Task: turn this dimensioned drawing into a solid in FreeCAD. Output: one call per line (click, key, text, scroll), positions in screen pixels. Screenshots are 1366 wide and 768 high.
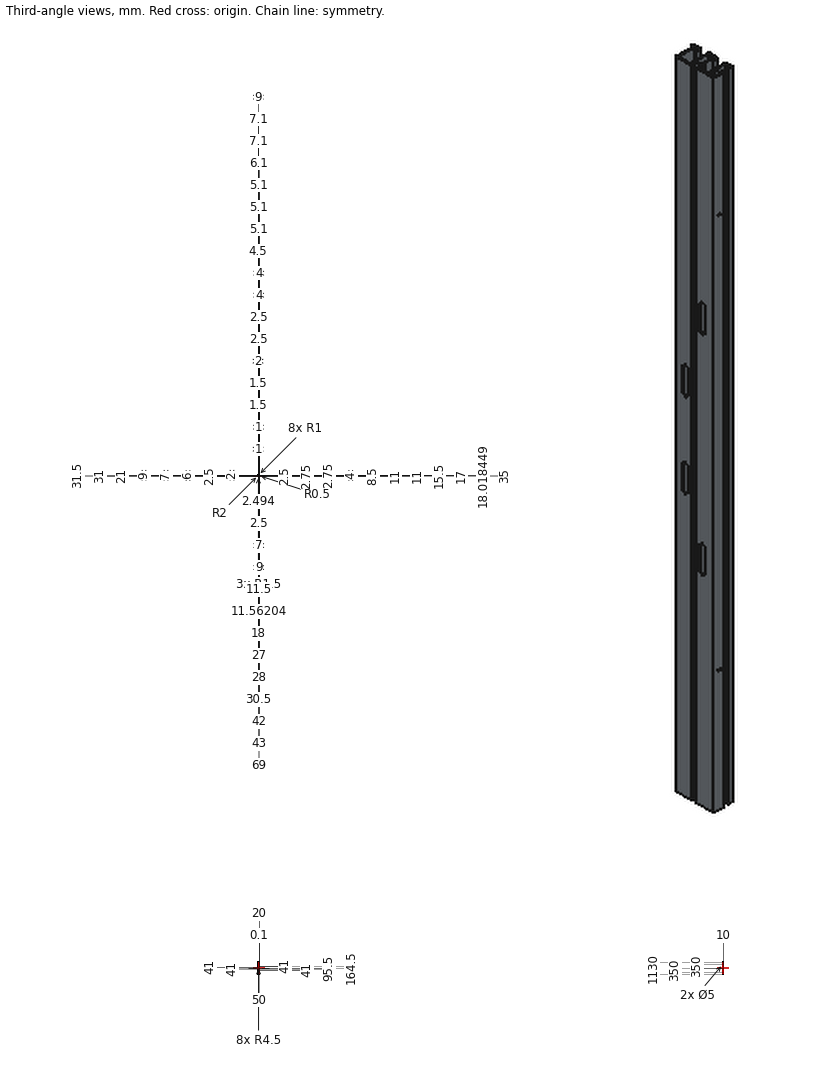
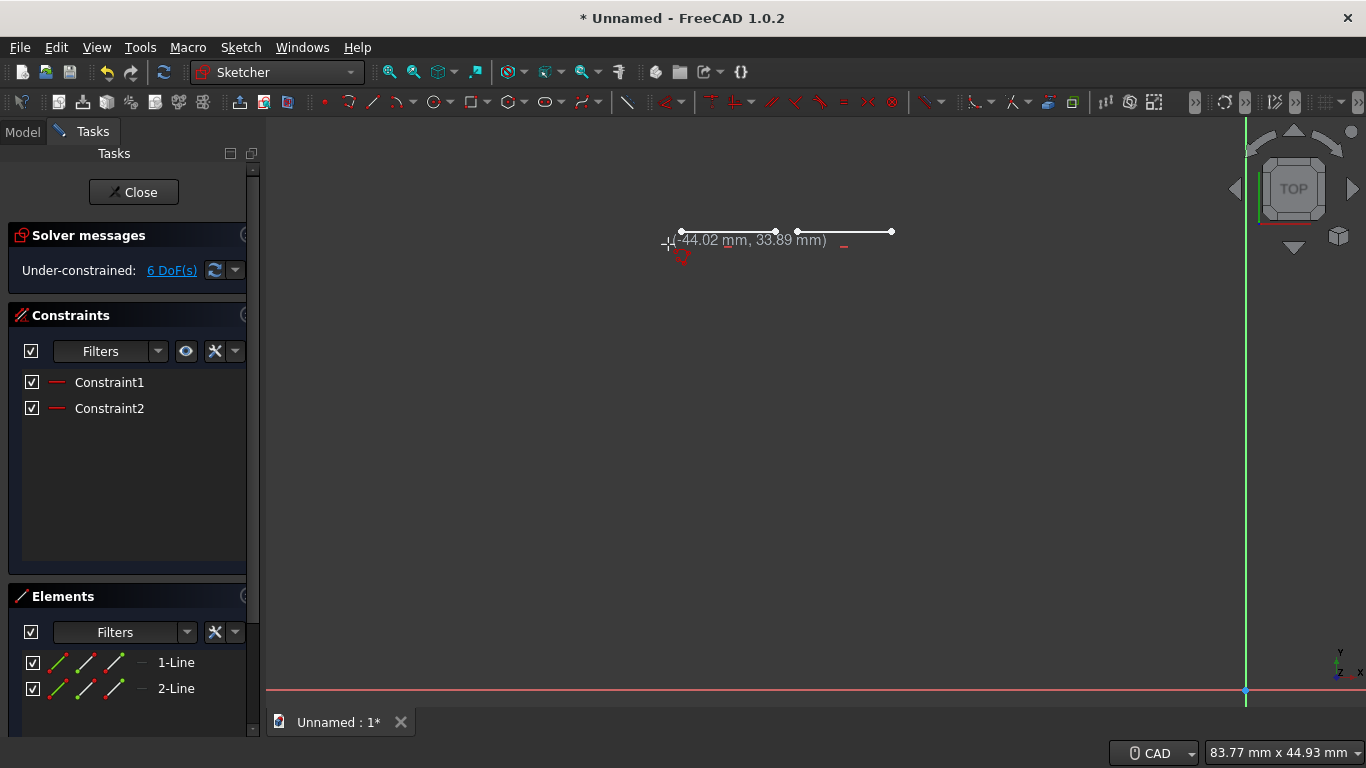
click(668, 244)
click(668, 658)
click(432, 658)
right_click(432, 658)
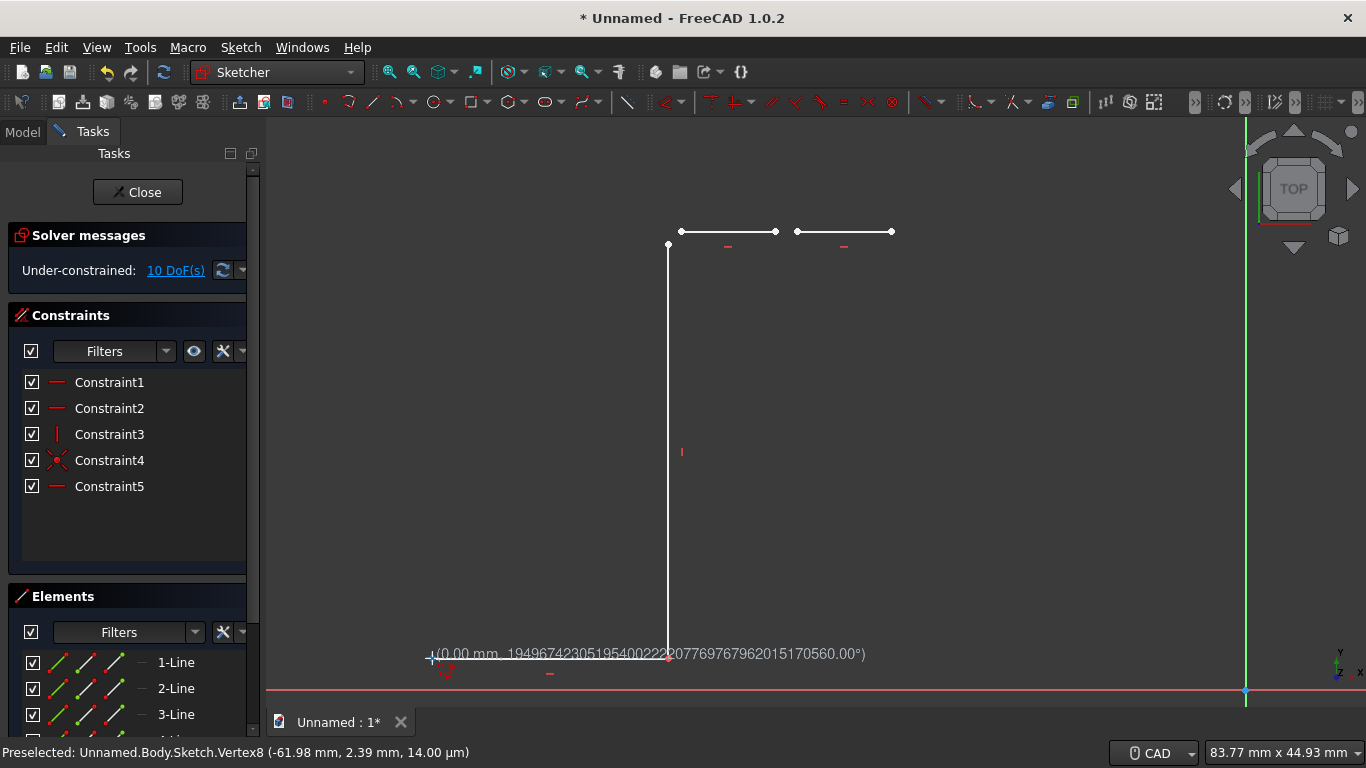
key(g)
key(l)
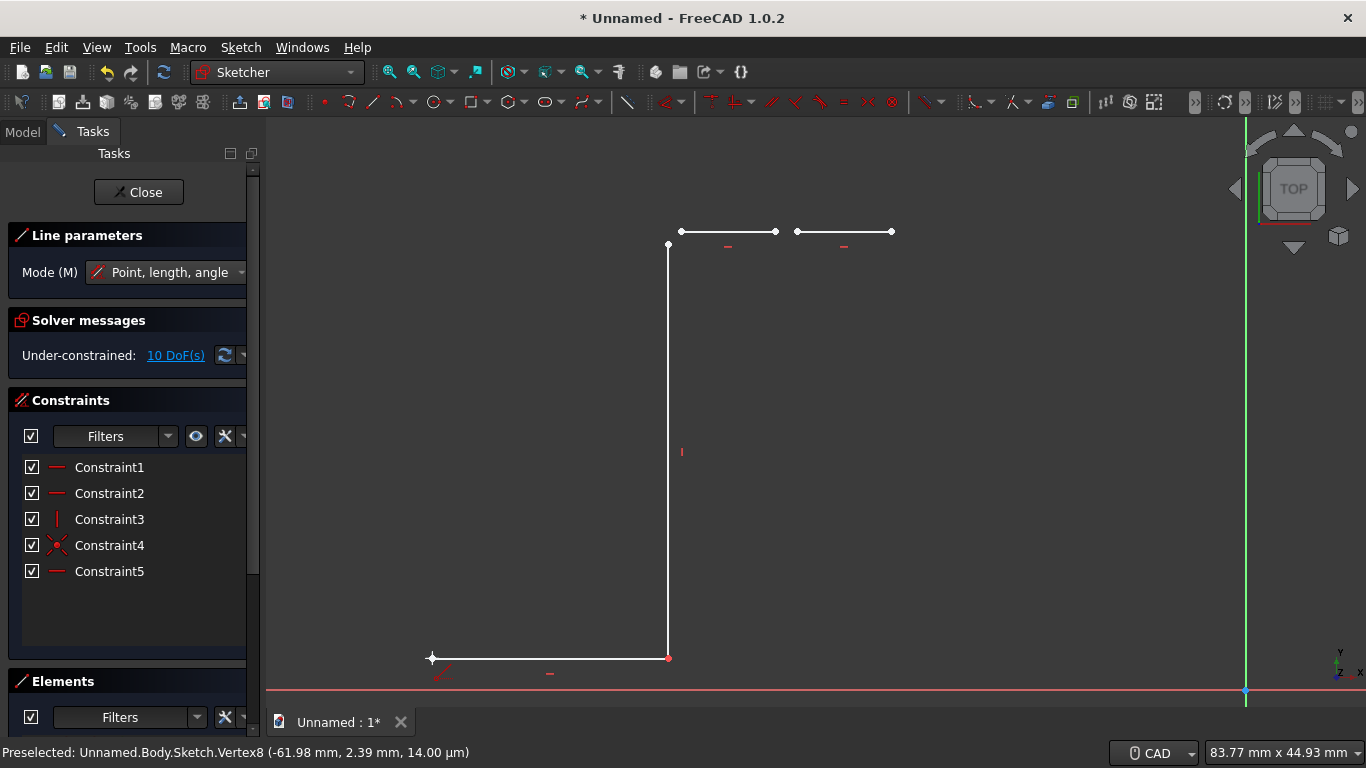
click(406, 631)
click(406, 283)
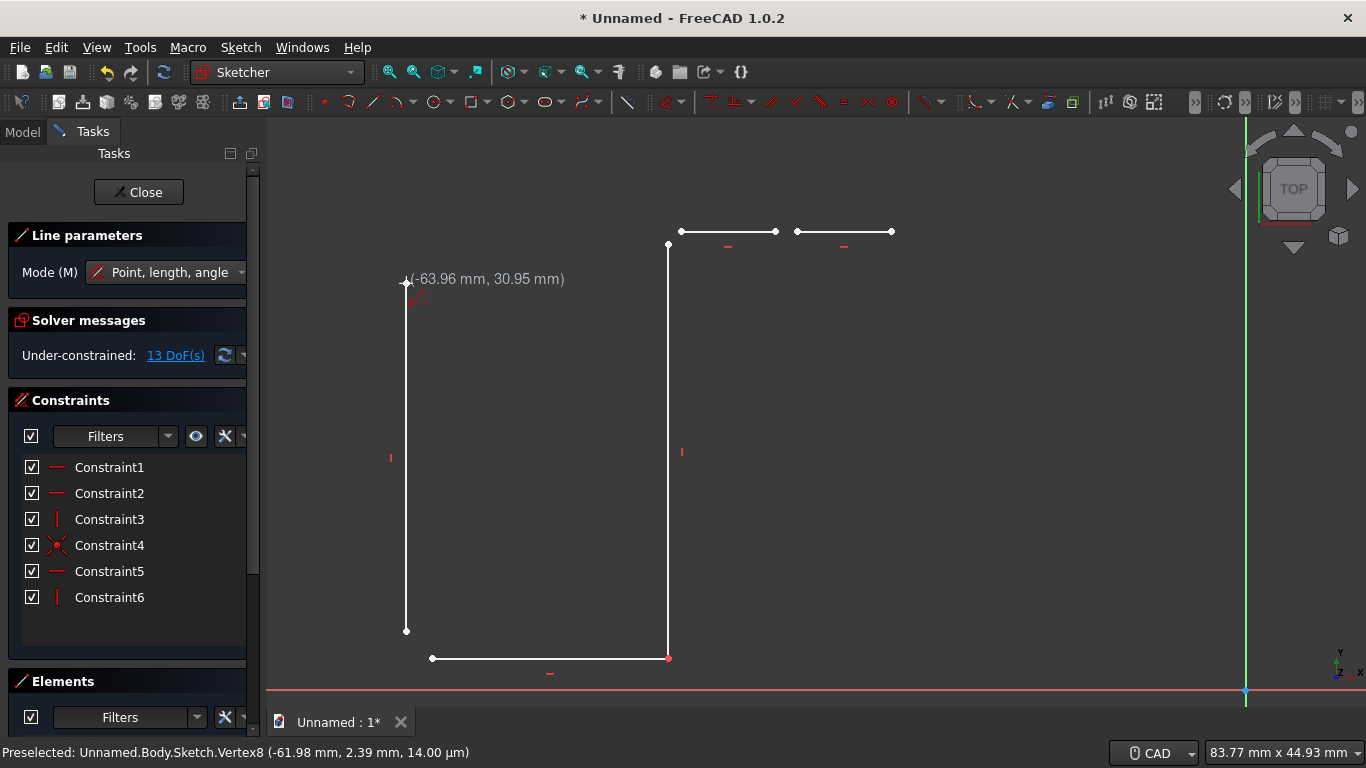
click(350, 102)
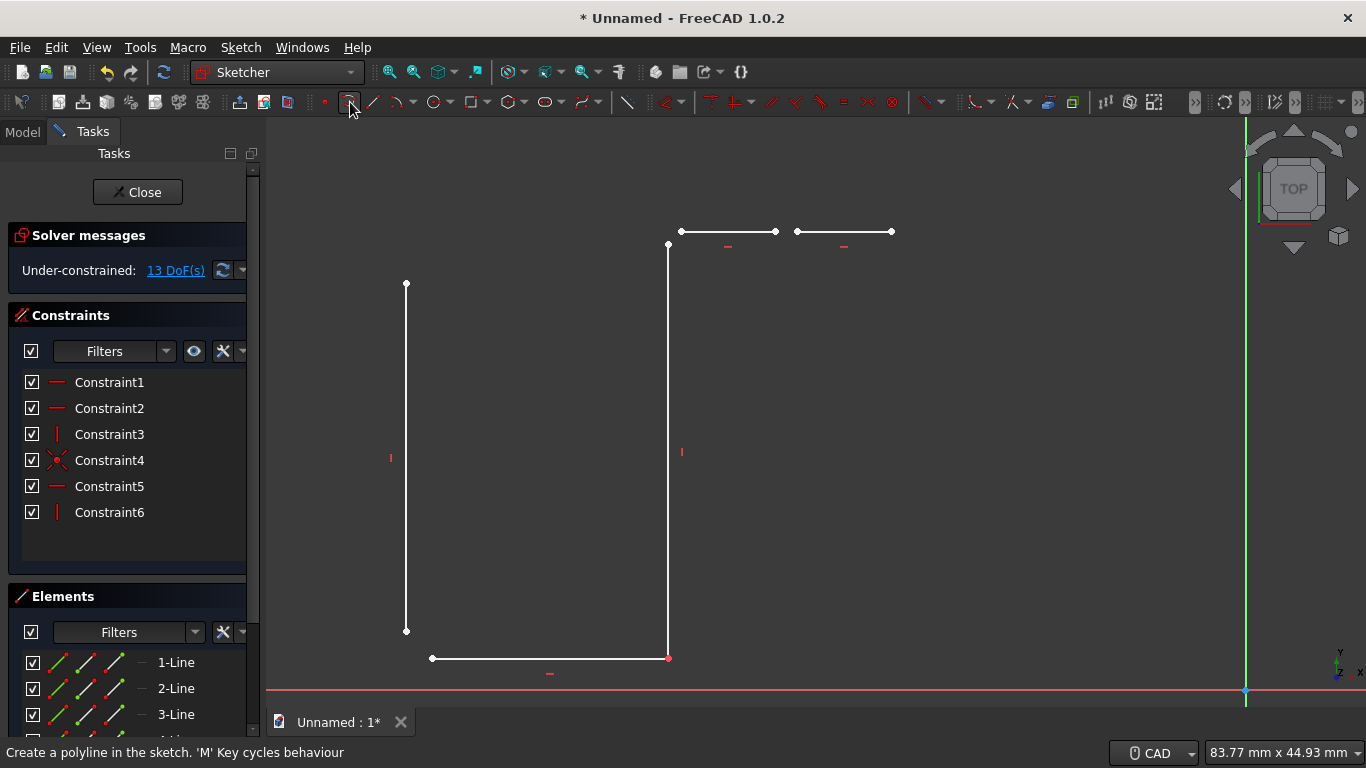
click(419, 270)
click(478, 270)
click(491, 362)
click(511, 362)
click(511, 244)
right_click(511, 244)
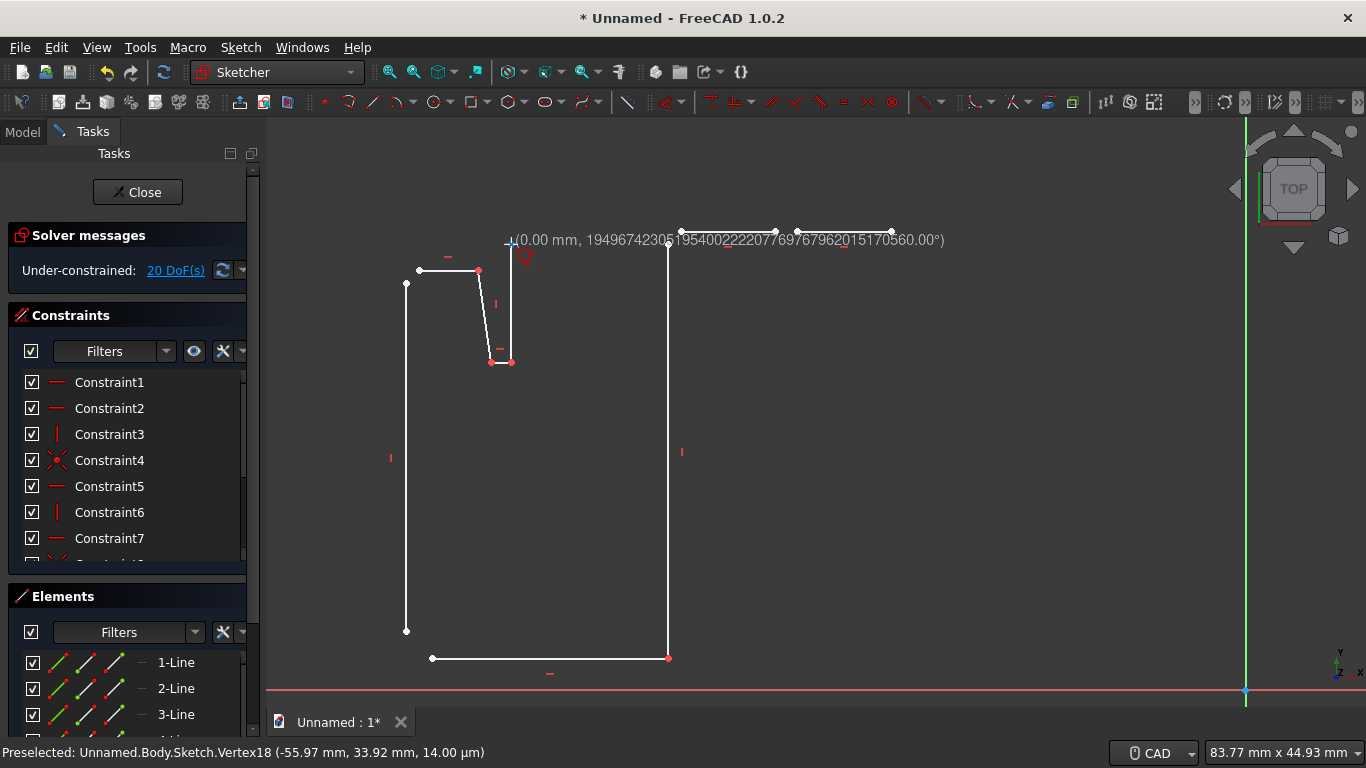
key(g)
key(l)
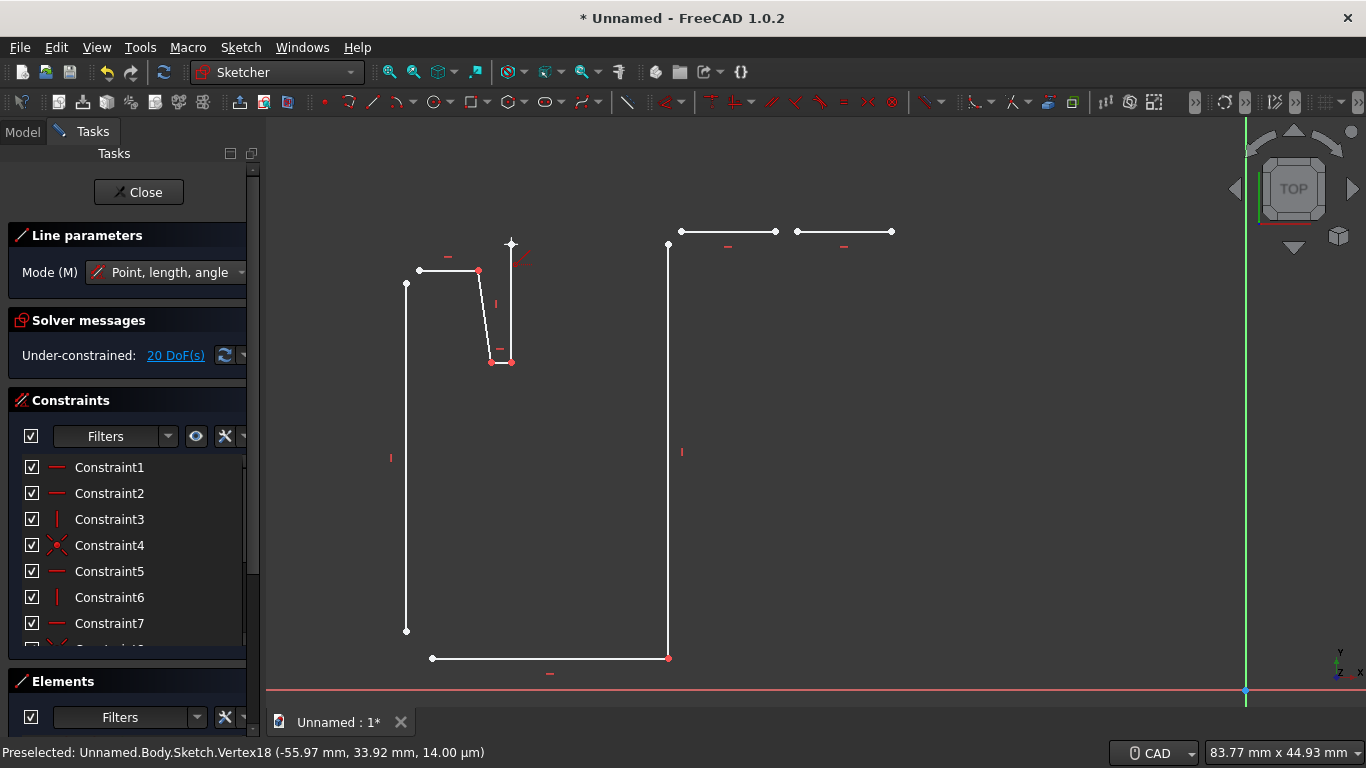
click(497, 231)
click(430, 231)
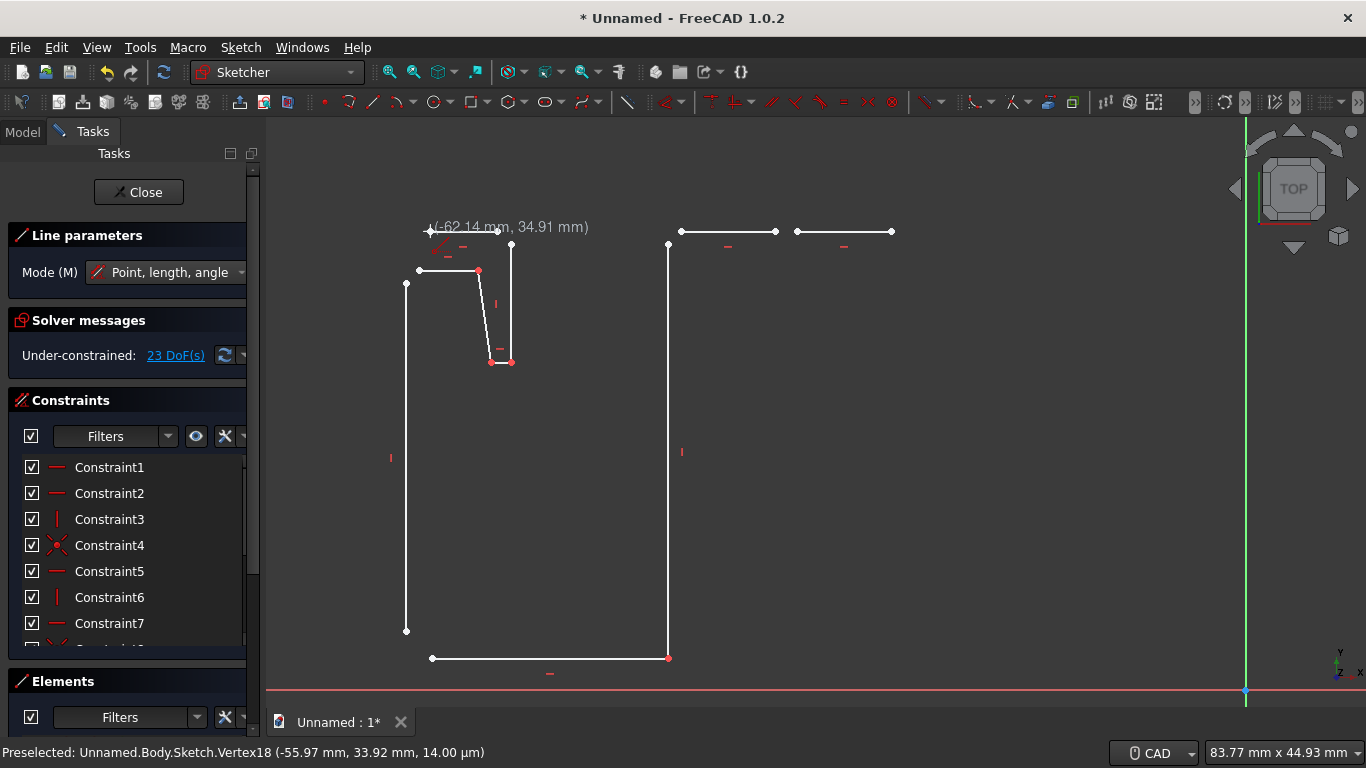
click(407, 231)
click(340, 231)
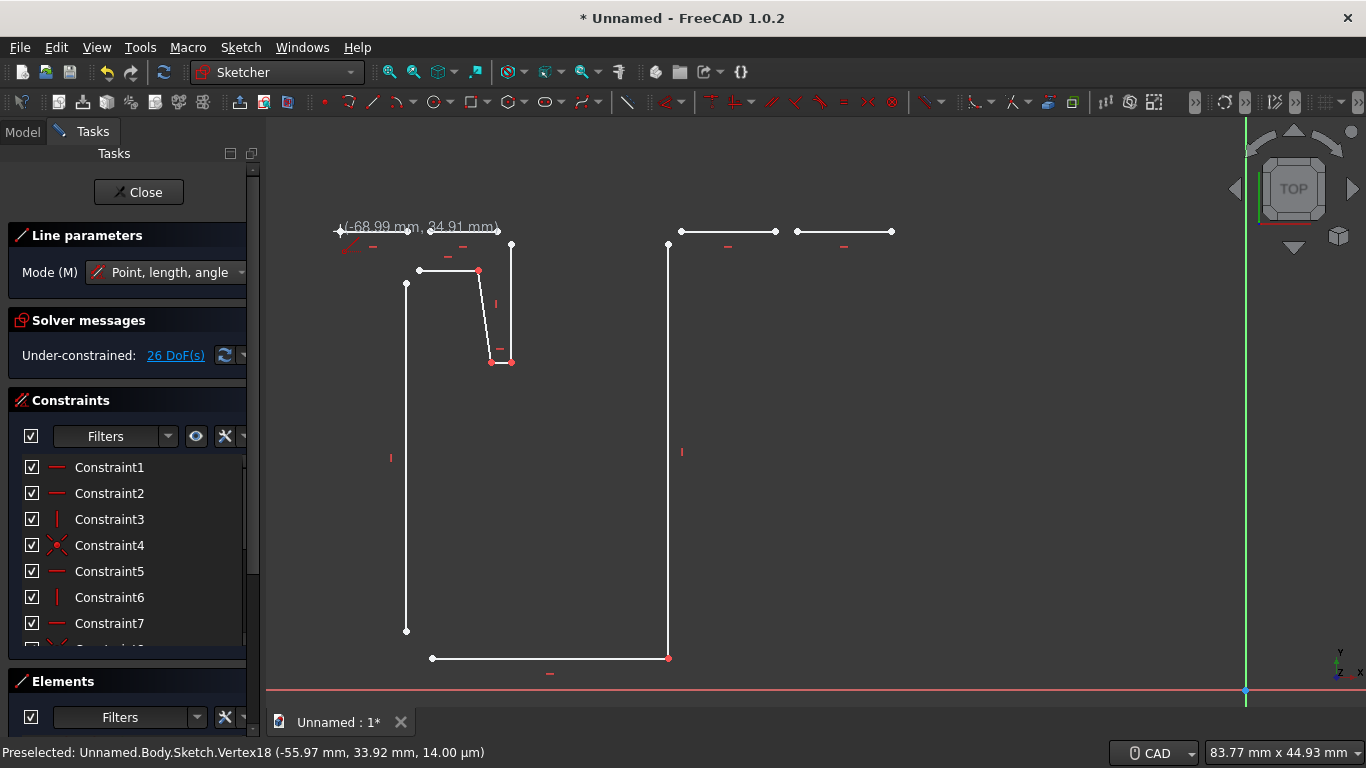
key(g)
key(m)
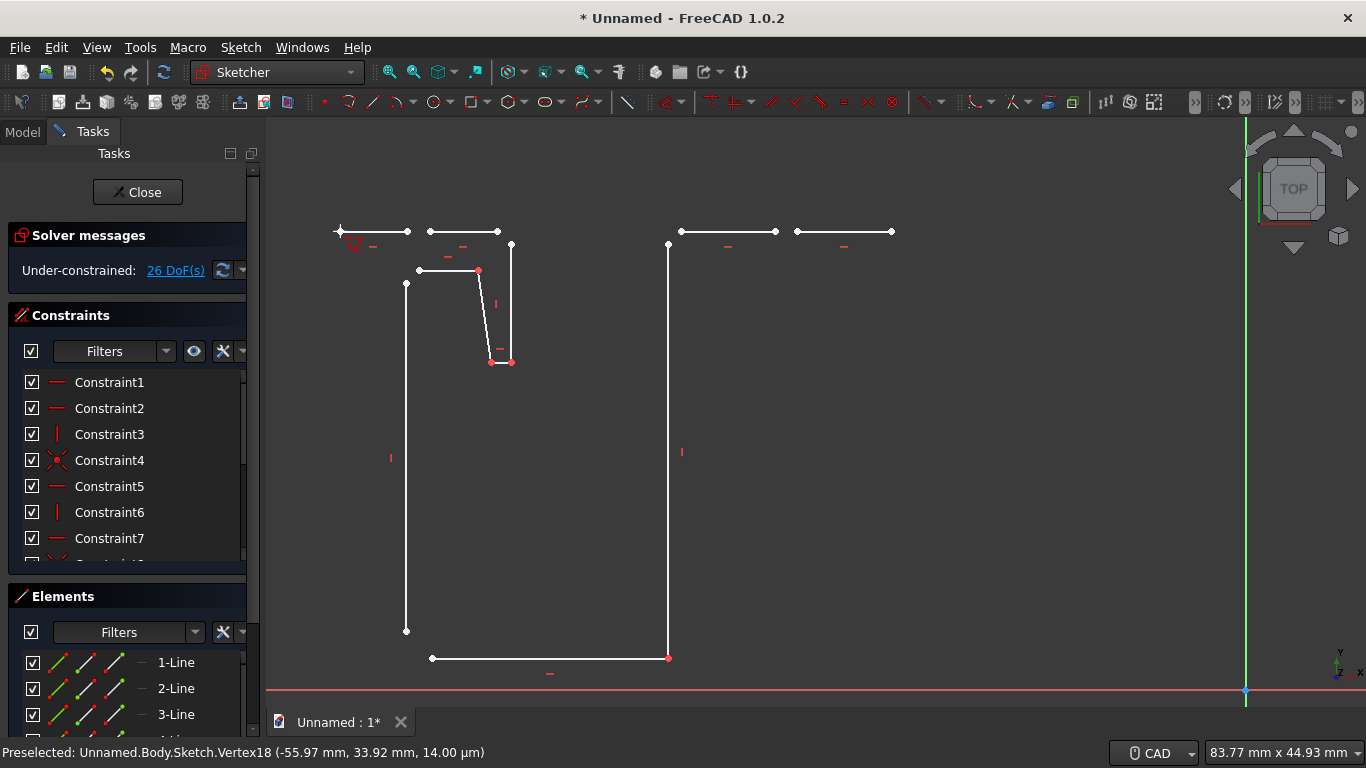
click(327, 244)
click(327, 270)
click(353, 270)
right_click(353, 270)